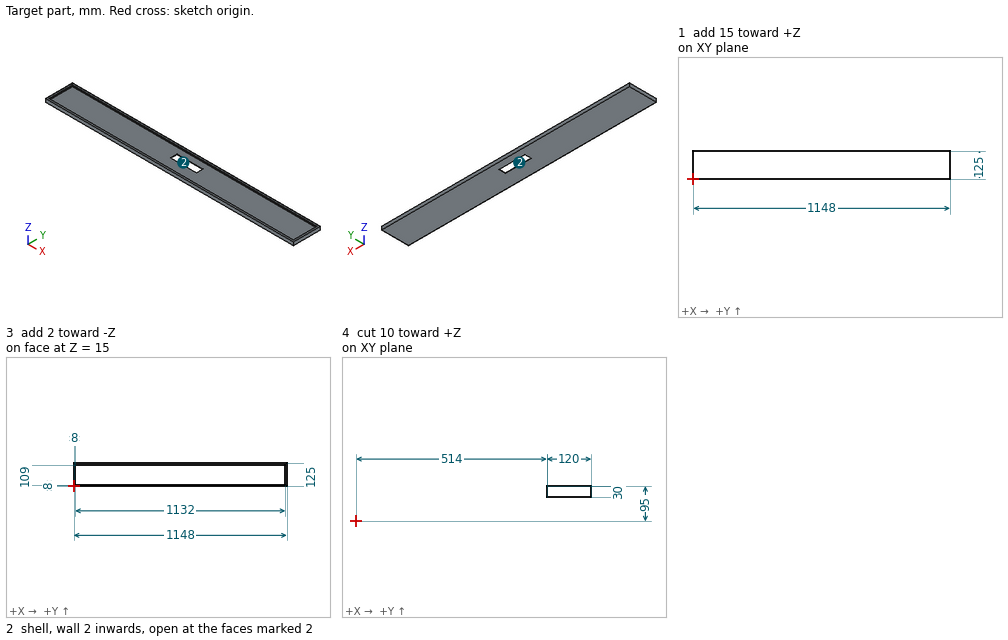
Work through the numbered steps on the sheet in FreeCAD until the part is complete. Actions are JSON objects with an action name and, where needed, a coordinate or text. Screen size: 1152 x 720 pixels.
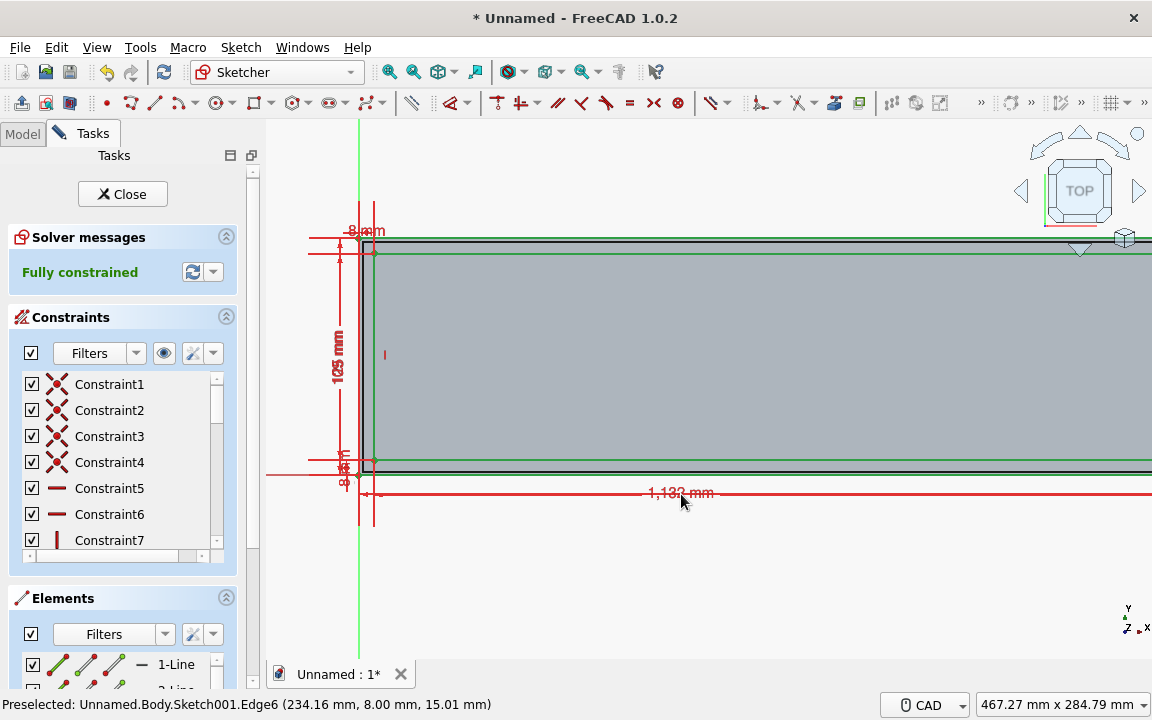
{"action": "left_click", "coordinate": [123, 194]}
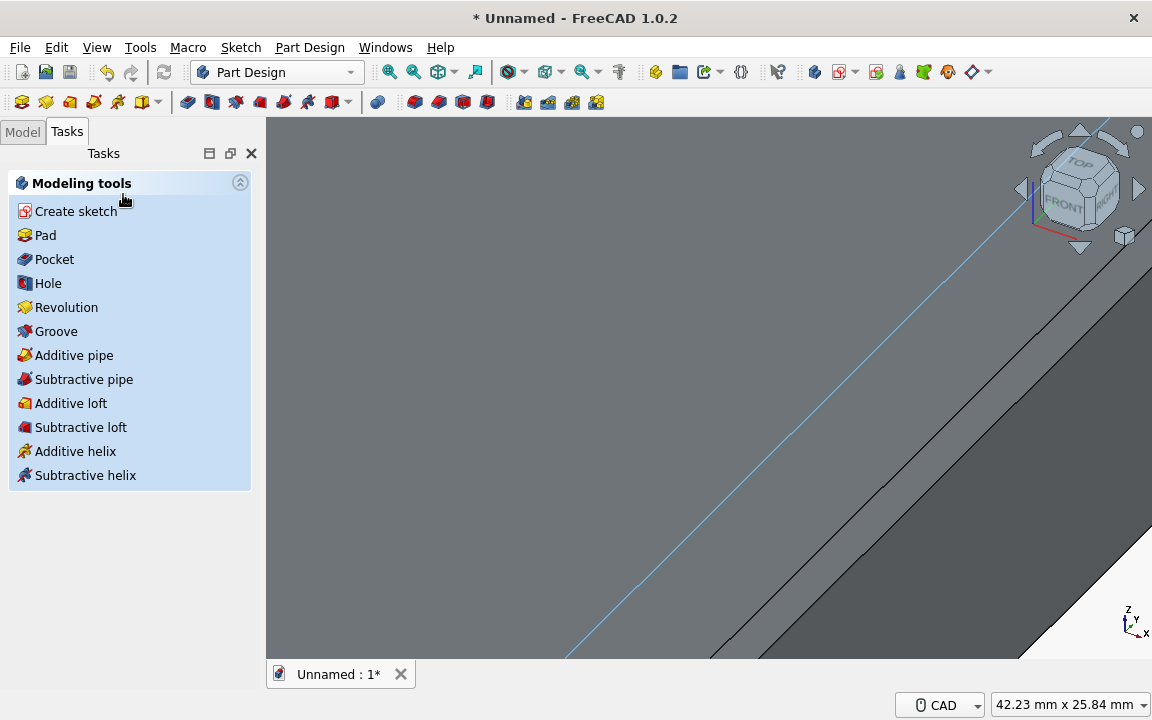
{"action": "left_click", "coordinate": [22, 102]}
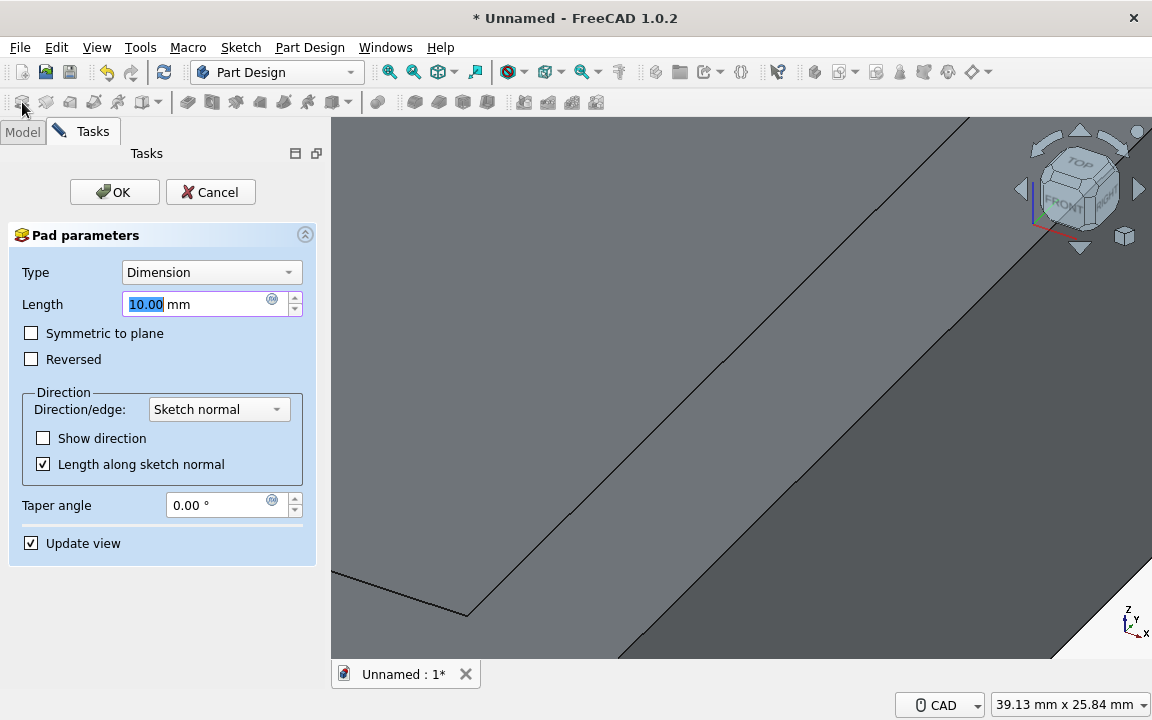
{"action": "type", "text": "2"}
{"action": "key", "text": "Tab"}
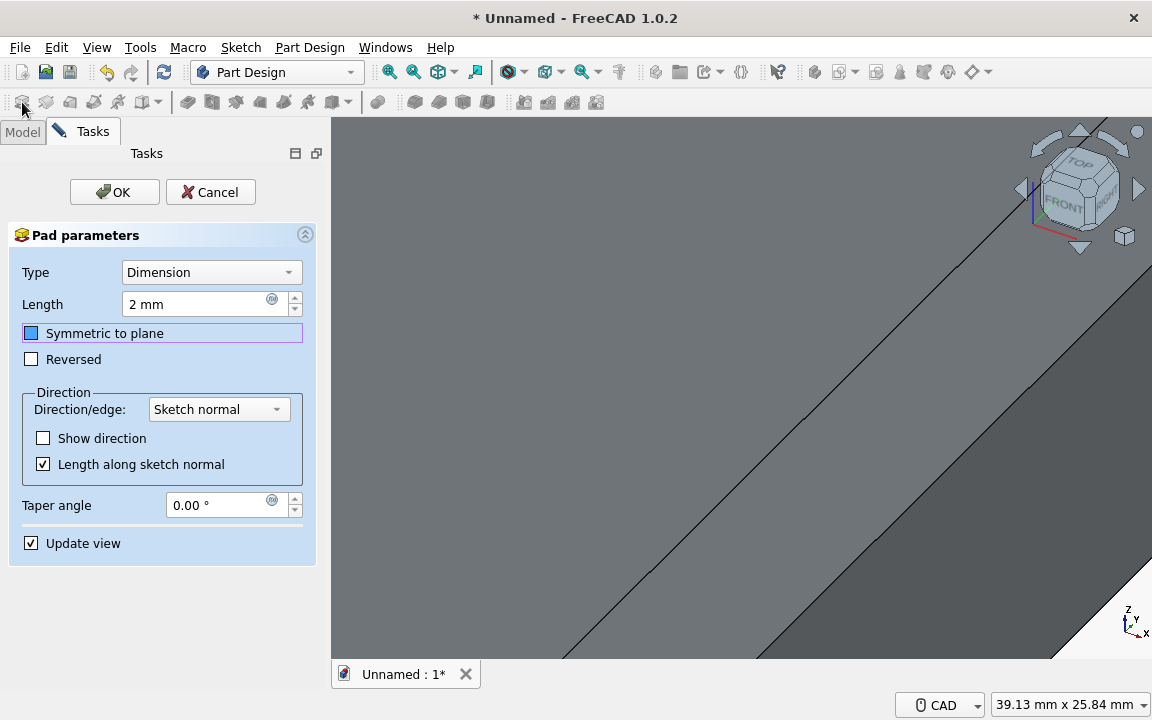
{"action": "left_click", "coordinate": [30, 359]}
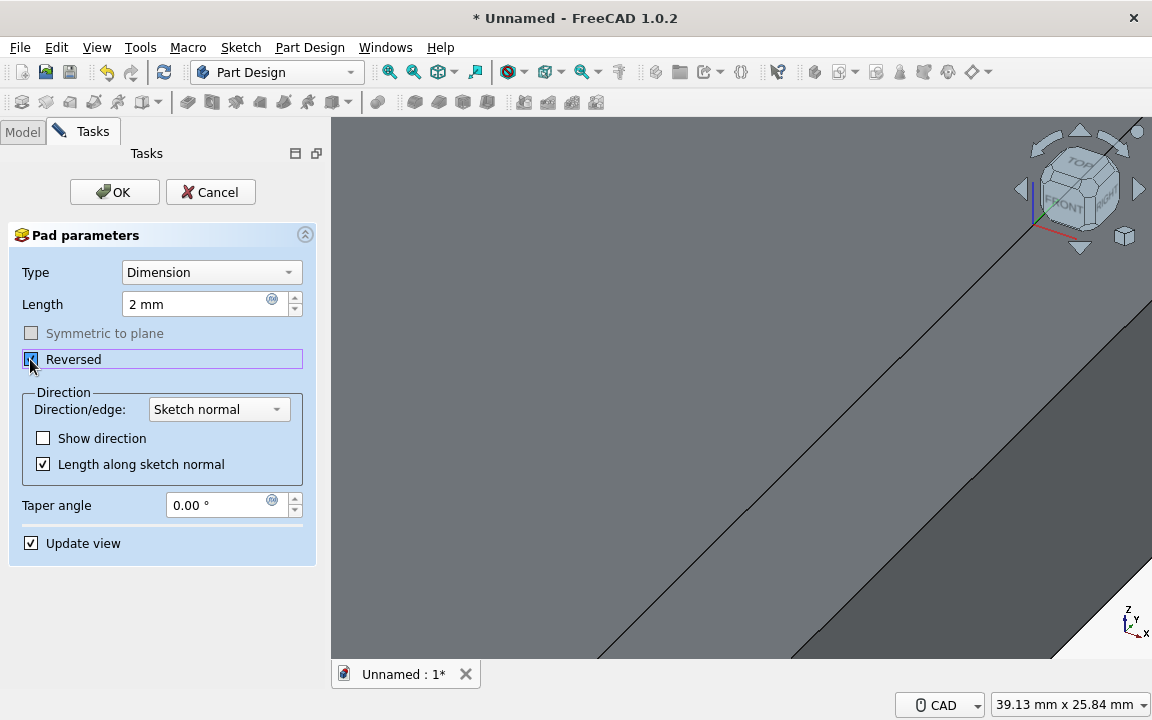
{"action": "left_click", "coordinate": [115, 192]}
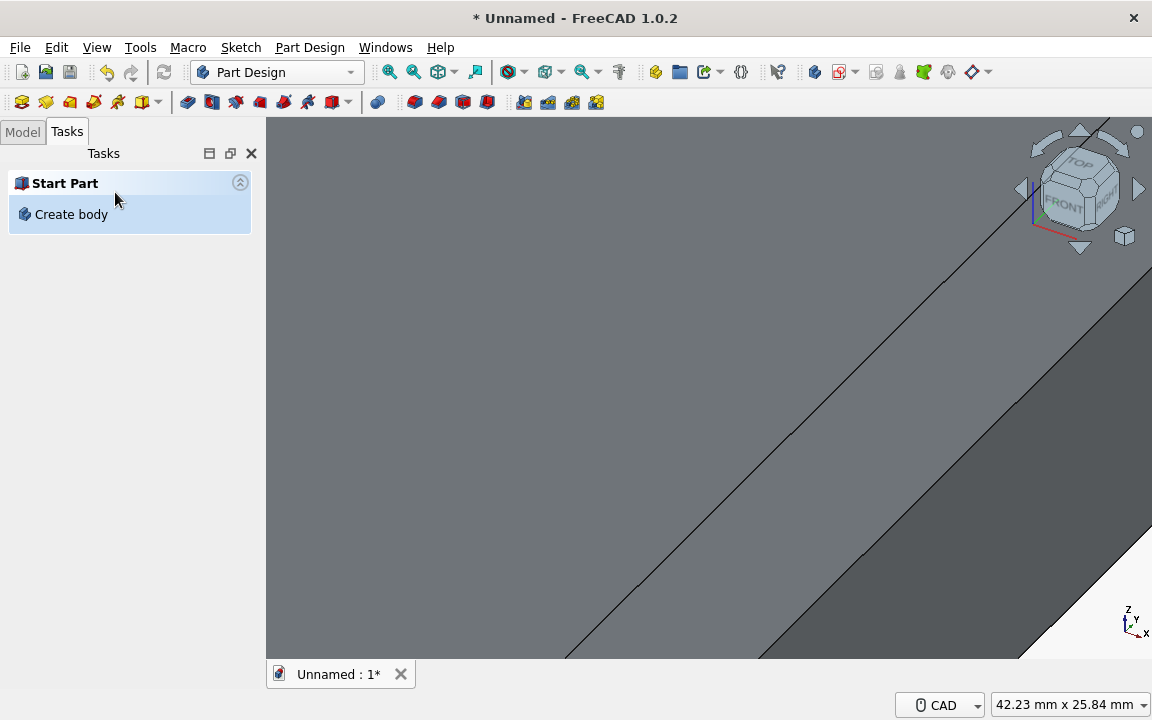
{"action": "left_click", "coordinate": [390, 72]}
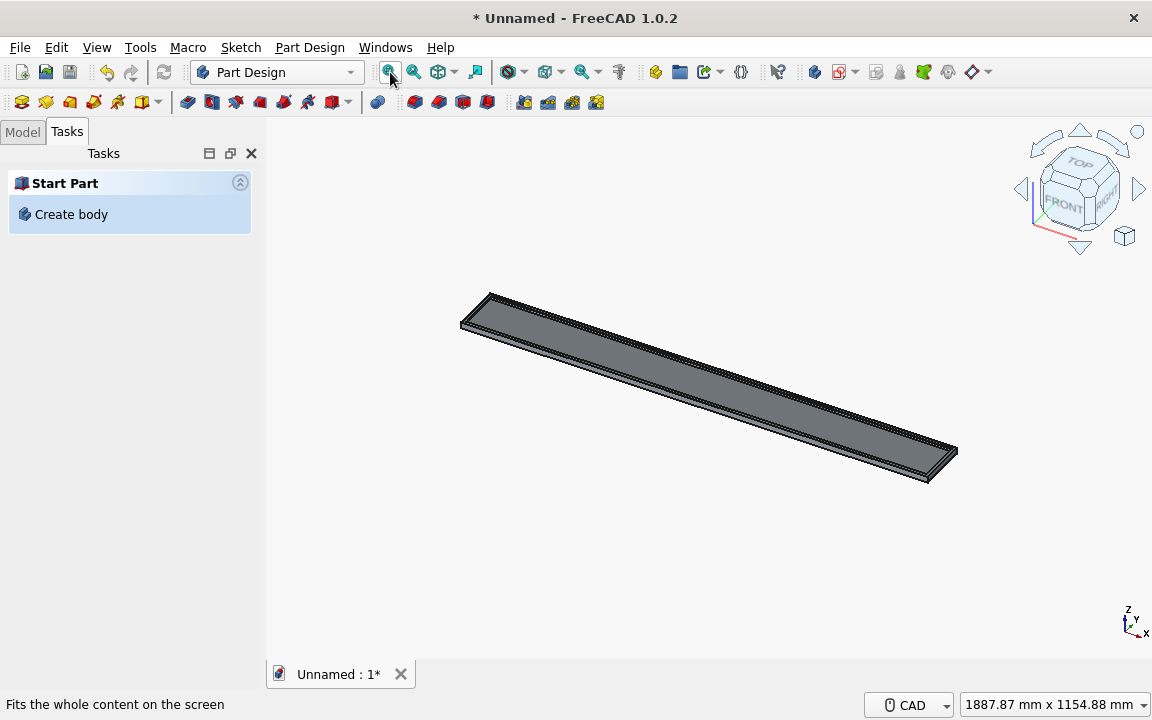
{"action": "left_click", "coordinate": [840, 72]}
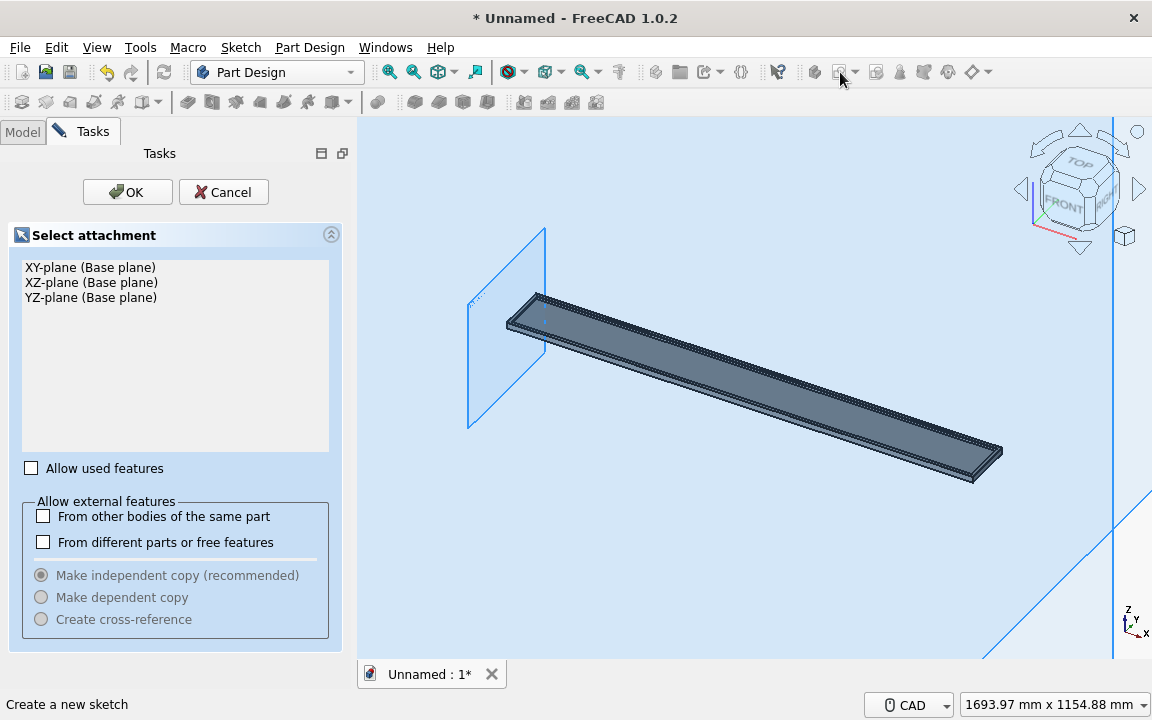
{"action": "left_click", "coordinate": [82, 268]}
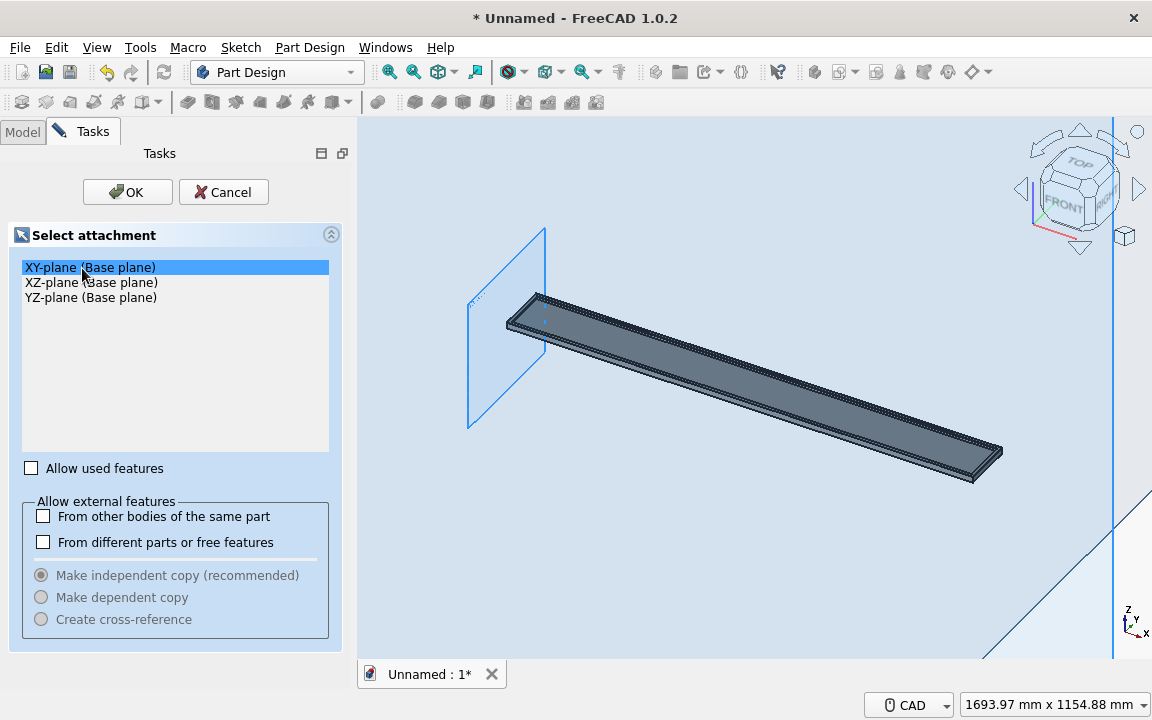
{"action": "left_click", "coordinate": [128, 192]}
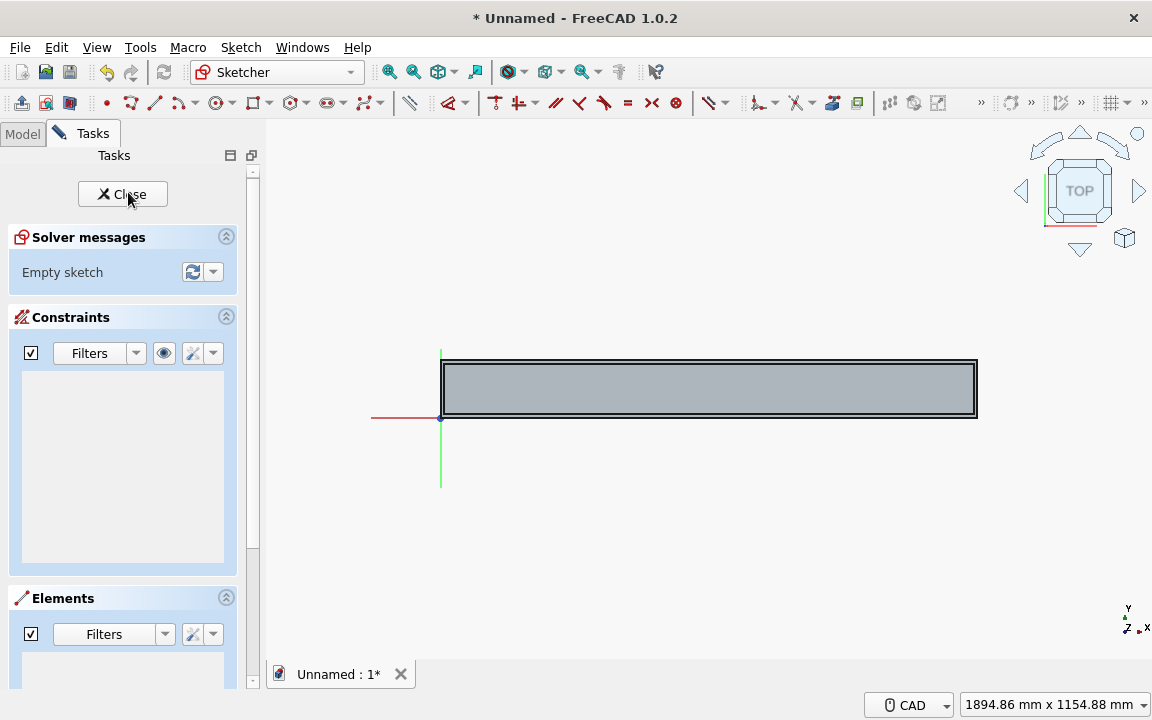
{"action": "left_click", "coordinate": [70, 104]}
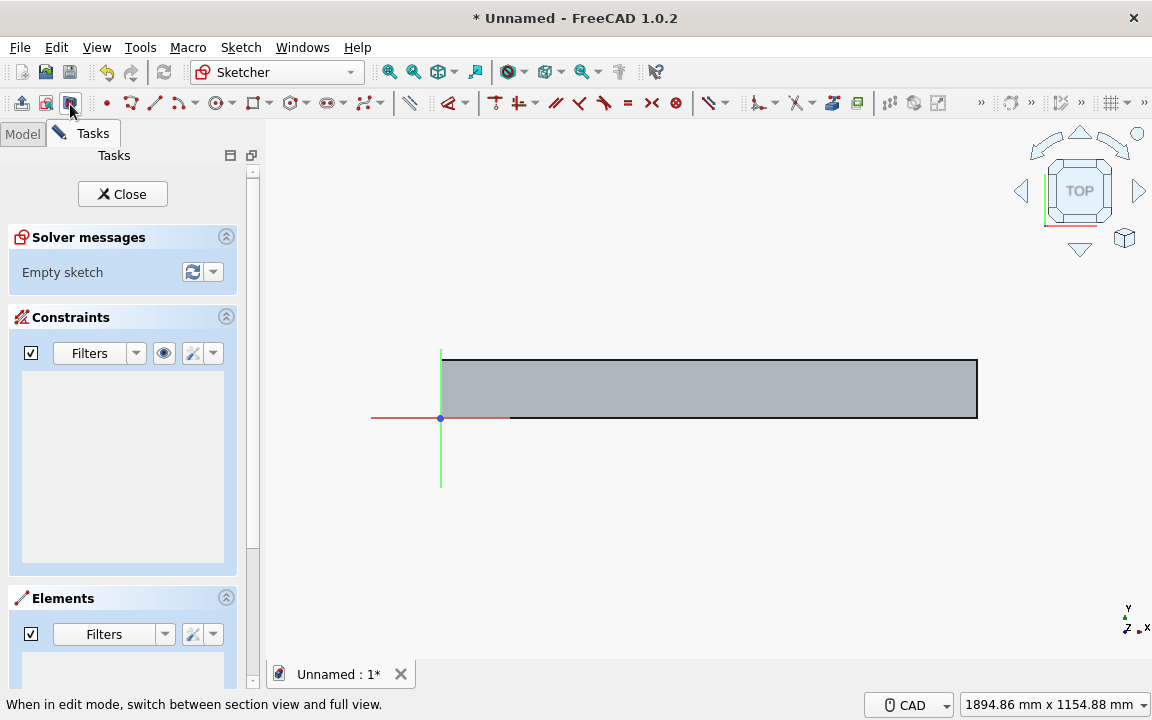
{"action": "scroll", "coordinate": [718, 380], "scroll_direction": "up", "scroll_amount": 11}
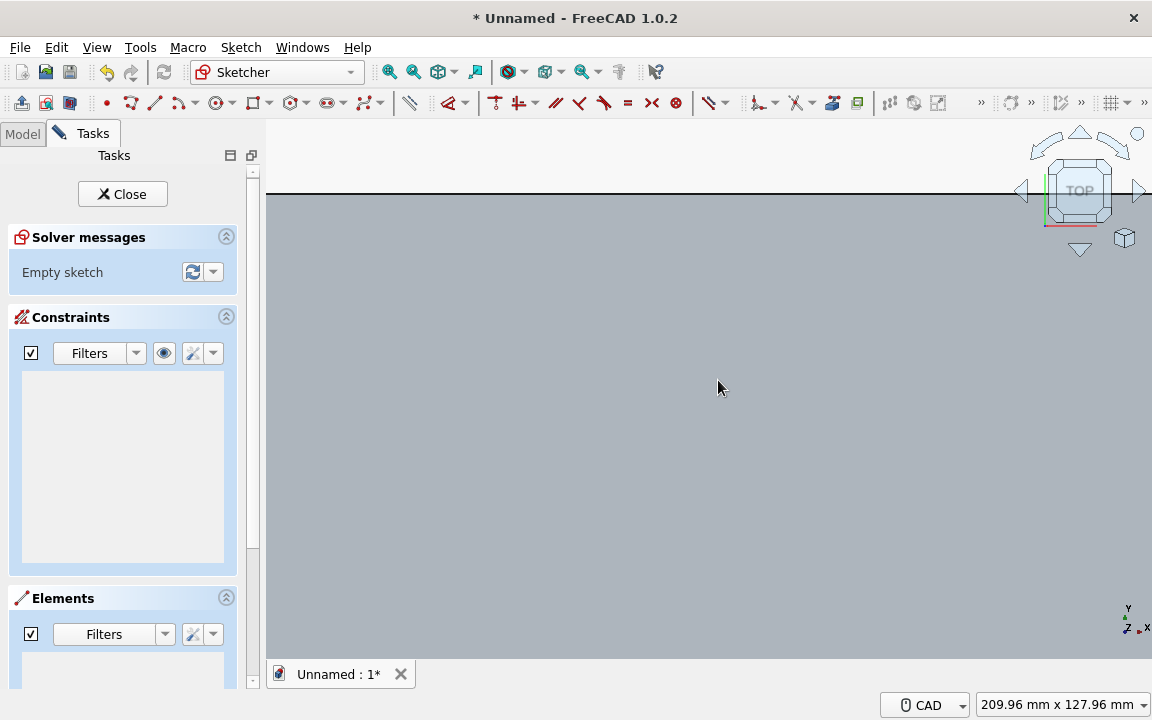
{"action": "left_click", "coordinate": [254, 104]}